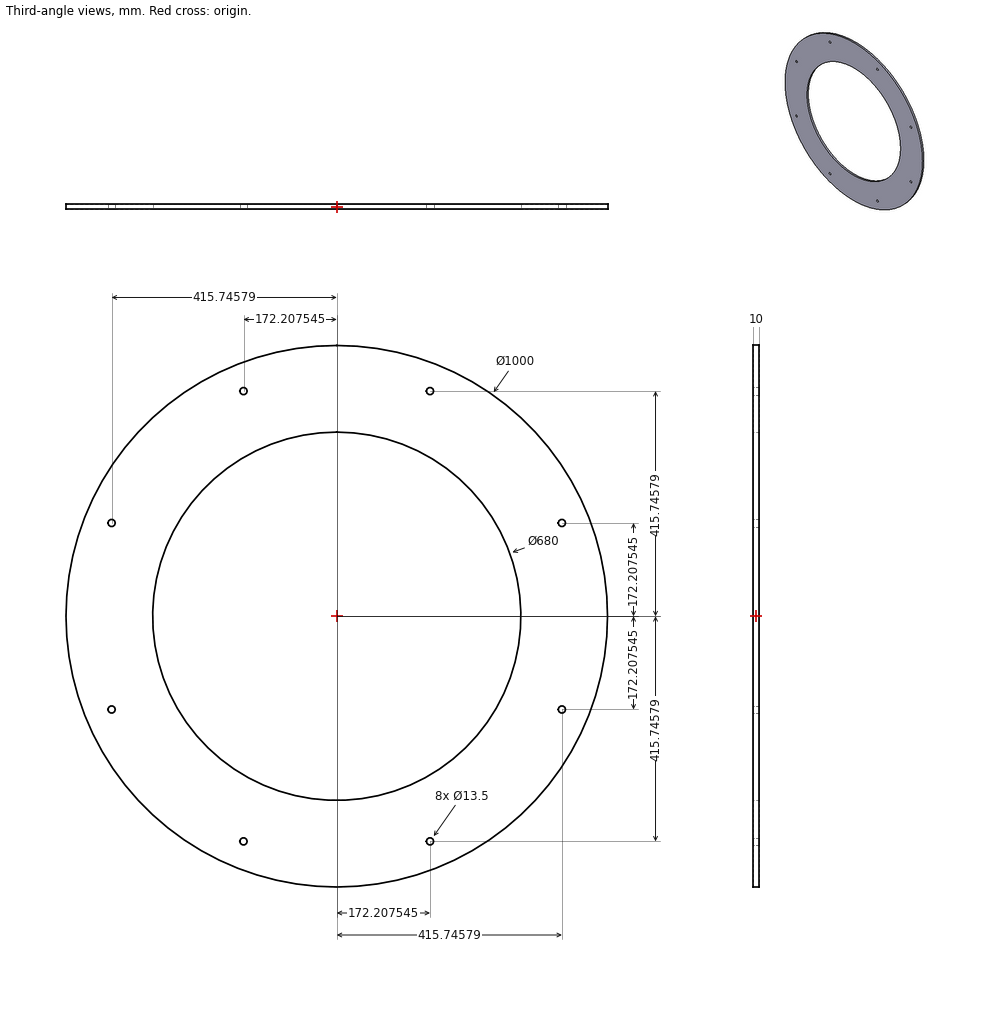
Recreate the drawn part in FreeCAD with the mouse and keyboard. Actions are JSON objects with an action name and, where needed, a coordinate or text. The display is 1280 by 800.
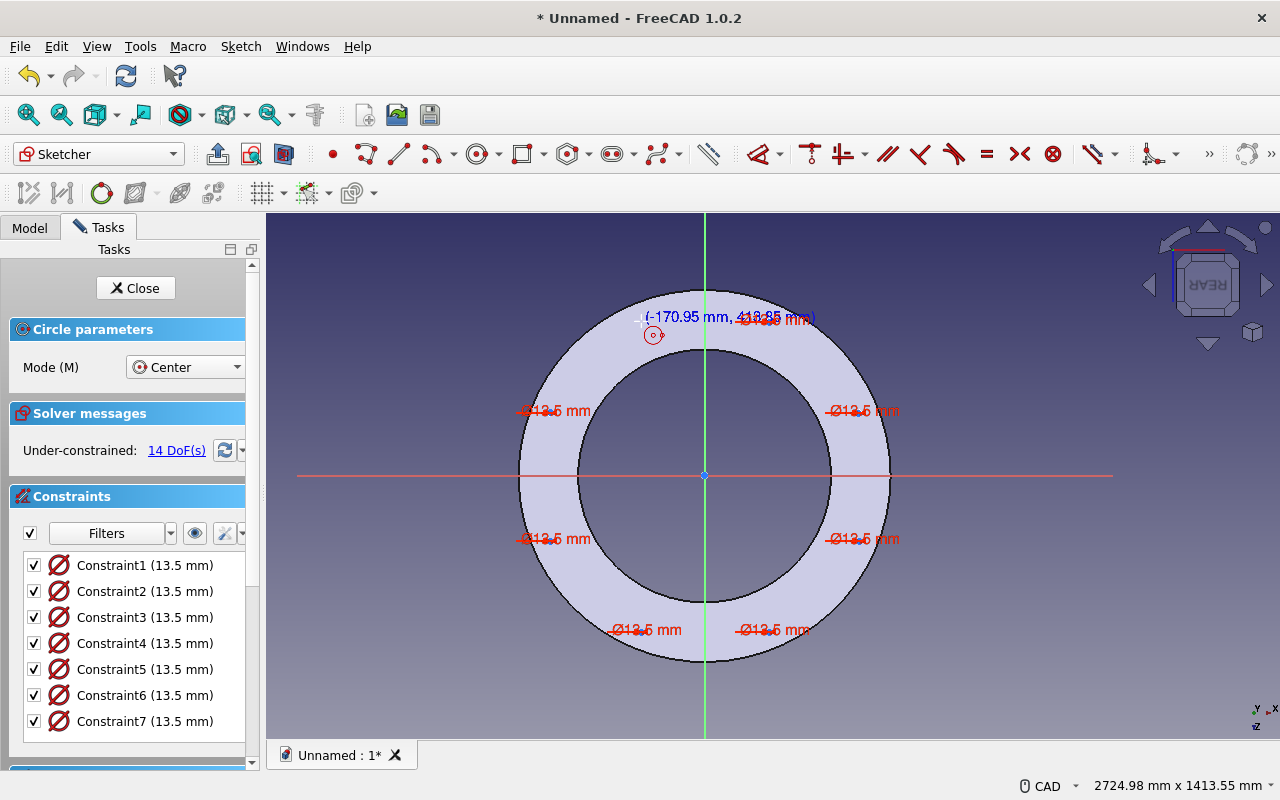
{"action": "left_click", "coordinate": [641, 321]}
{"action": "mouse_move", "coordinate": [642, 320]}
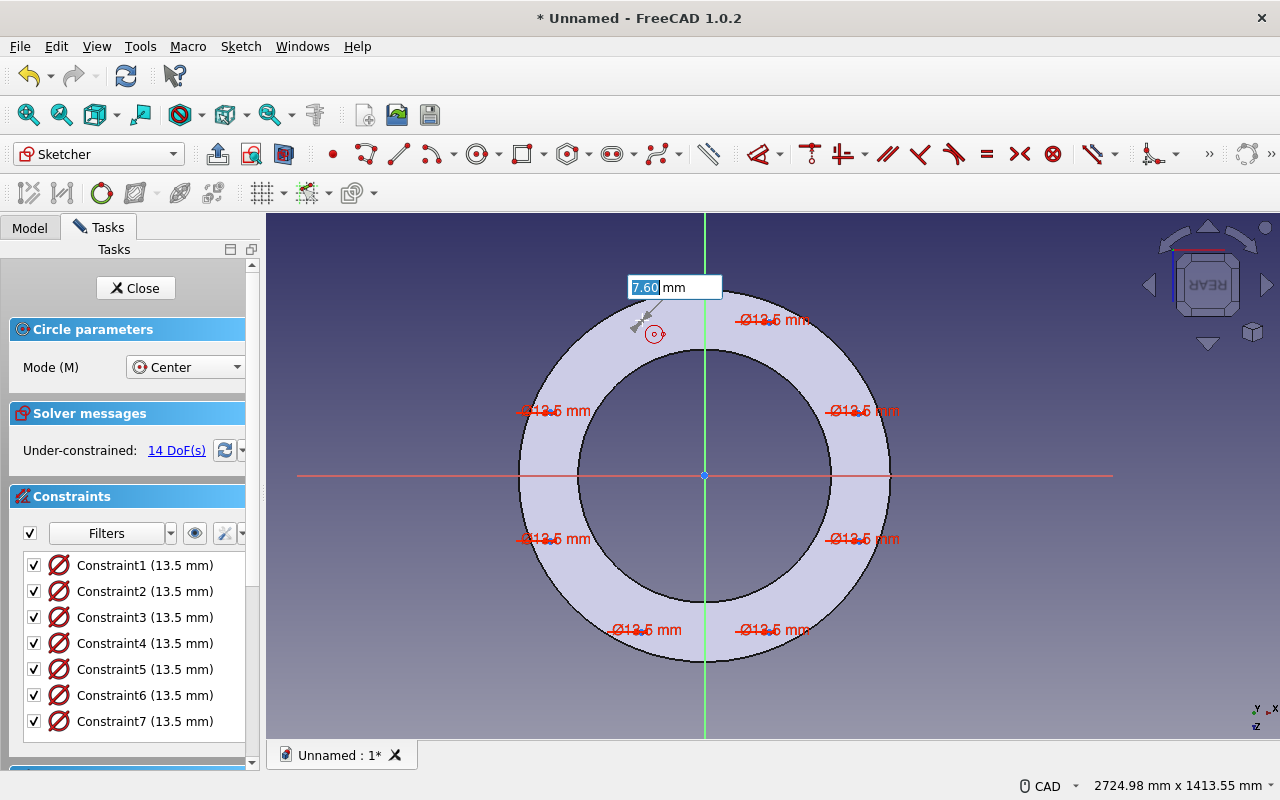
{"action": "type", "text": "13.5"}
{"action": "key", "text": "Return"}
{"action": "key", "text": "Escape"}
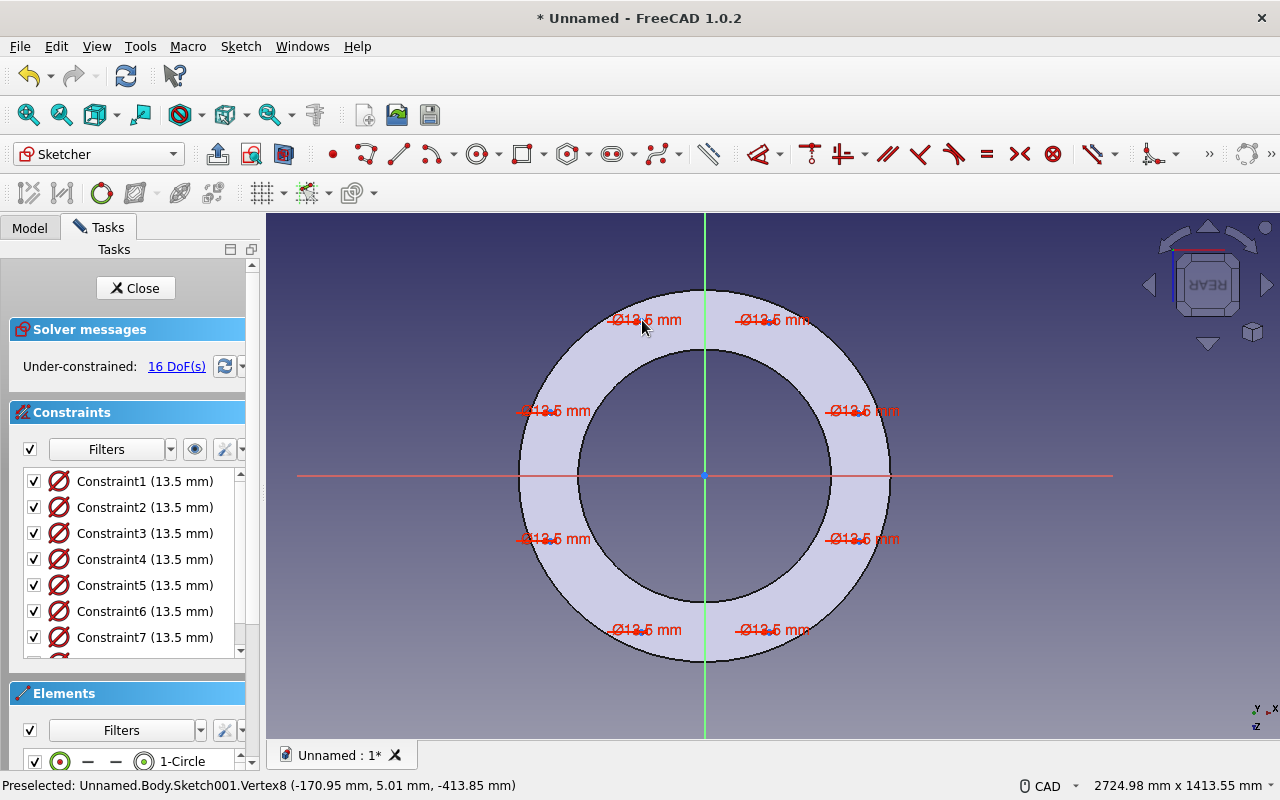
{"action": "left_click", "coordinate": [859, 413]}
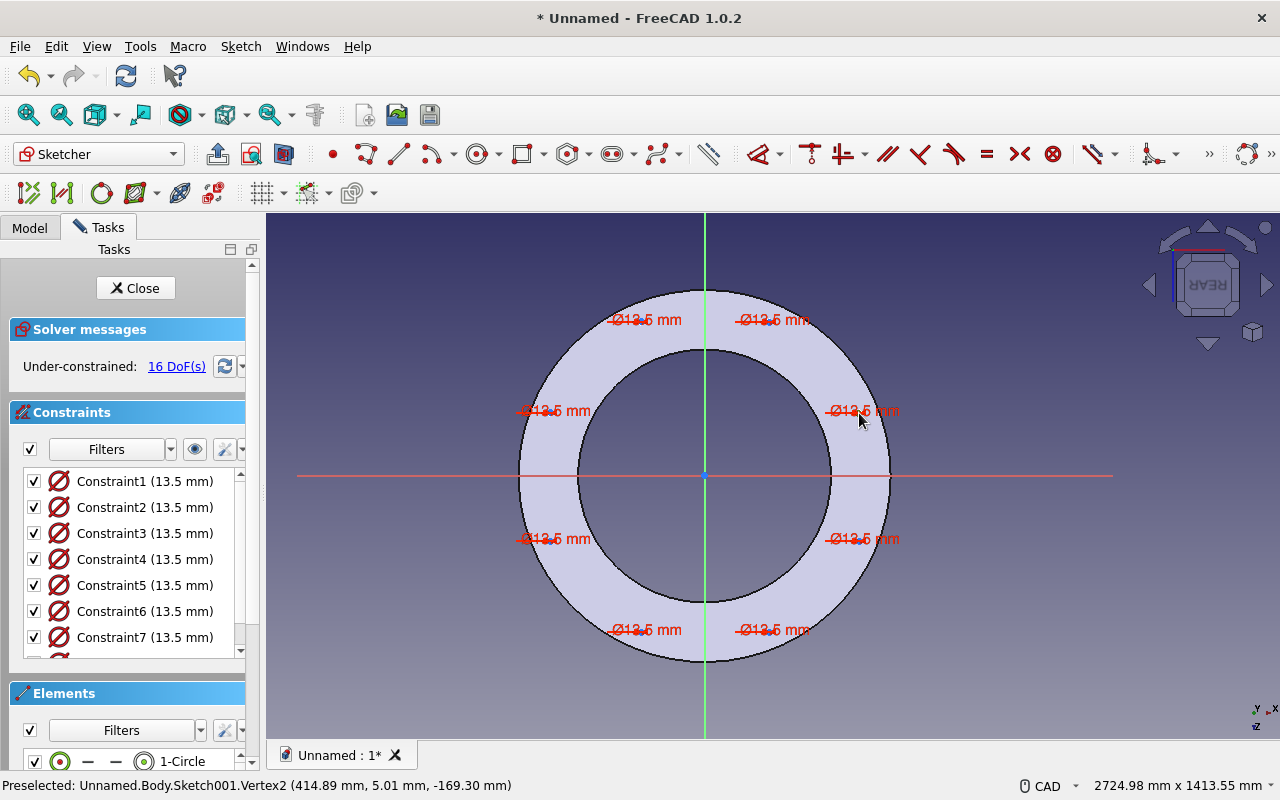
{"action": "left_click", "coordinate": [859, 541]}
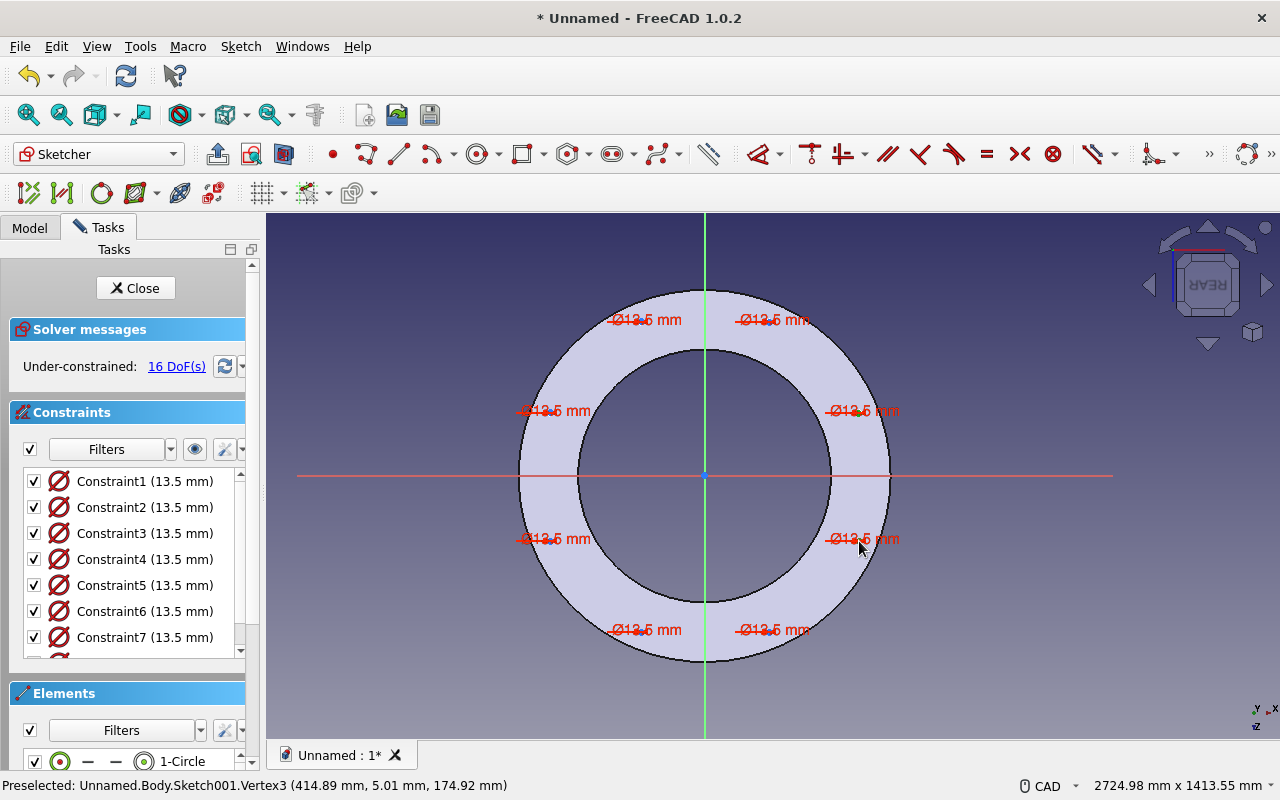
{"action": "key", "text": "v"}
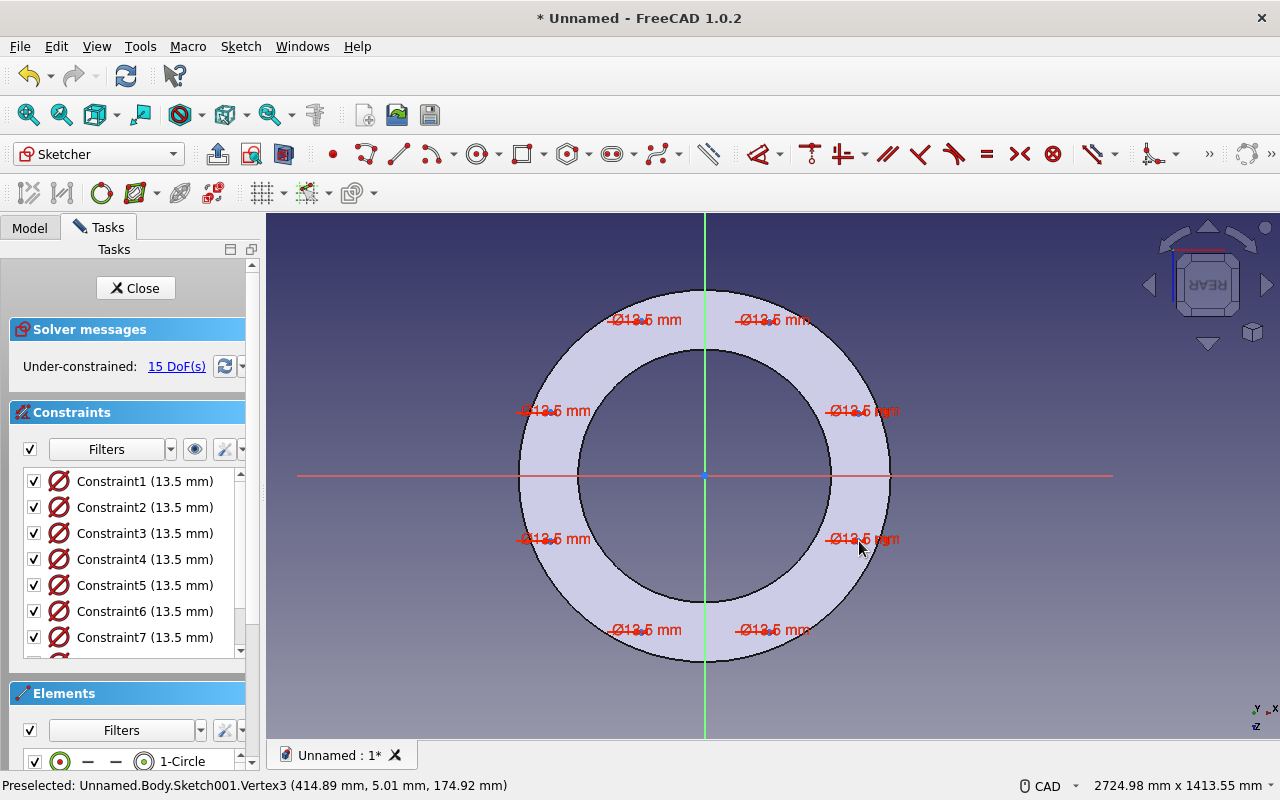
{"action": "left_click", "coordinate": [769, 322]}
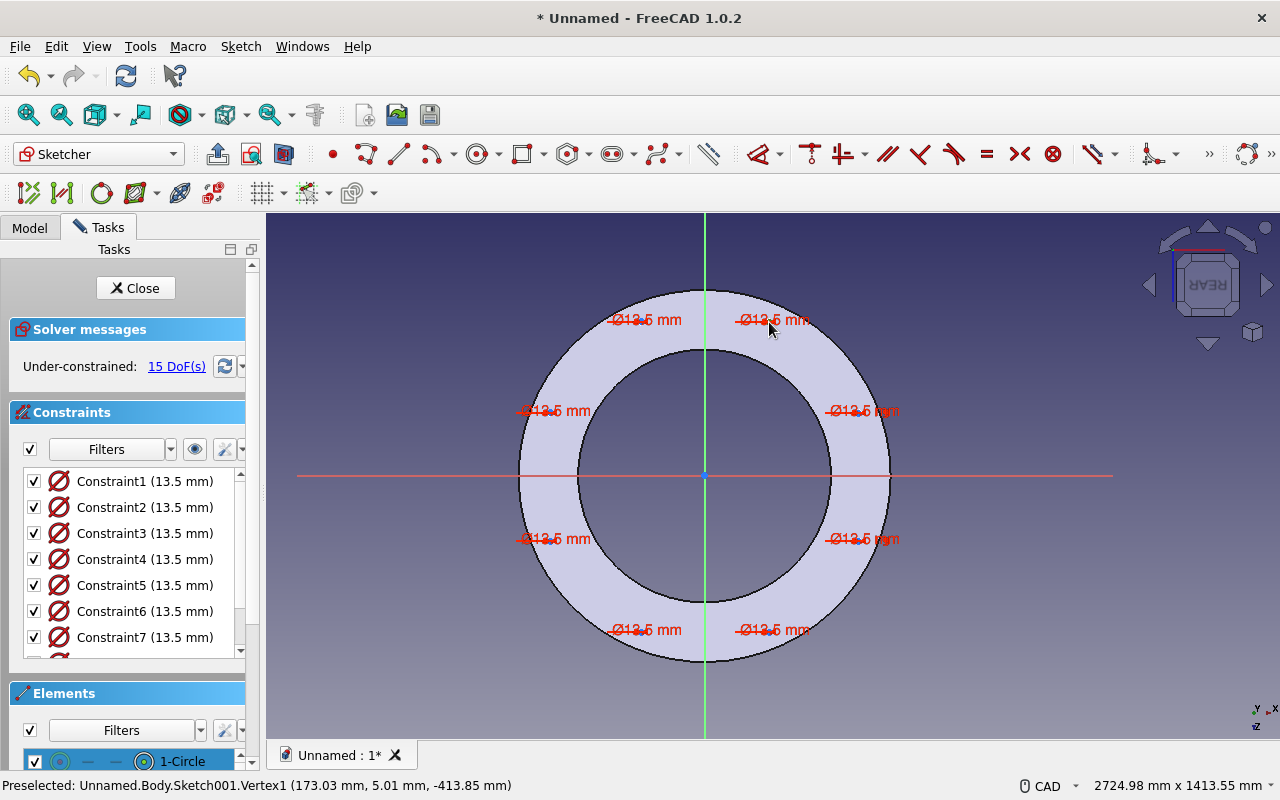
{"action": "left_click", "coordinate": [769, 632]}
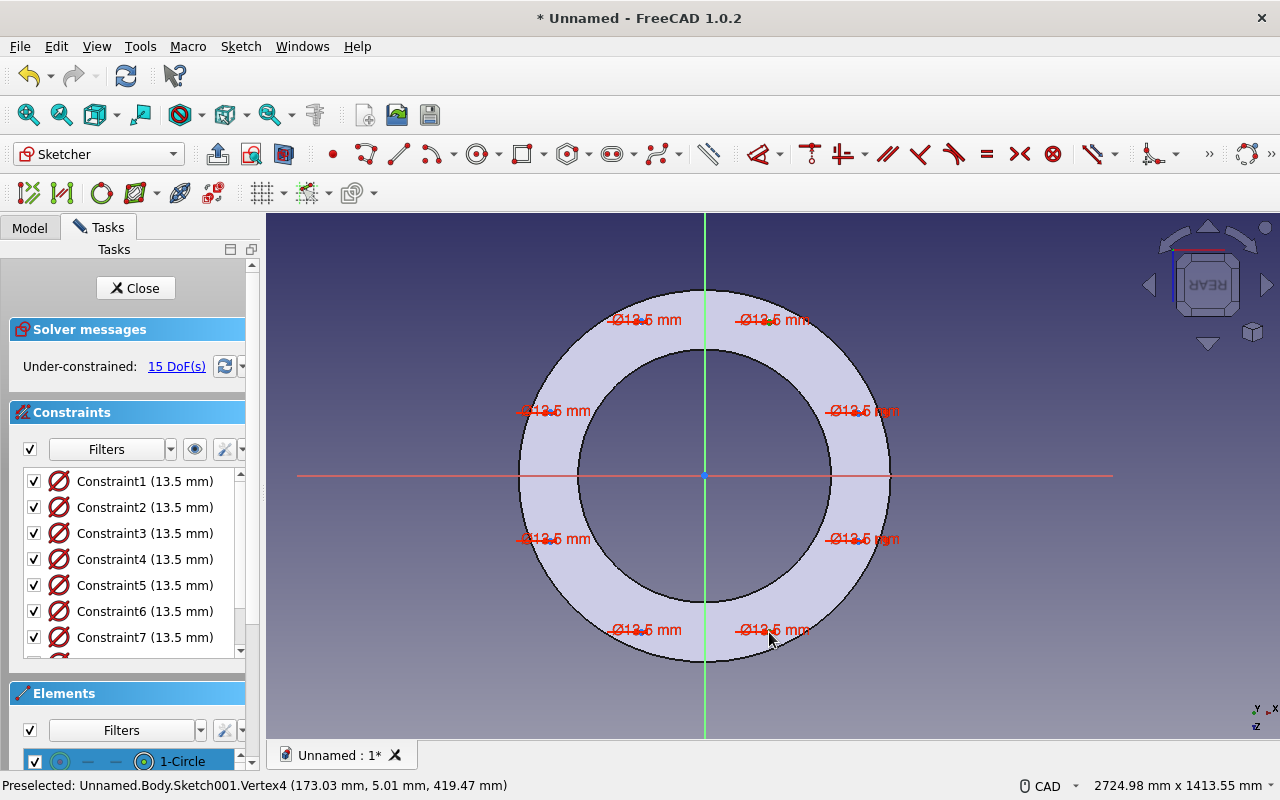
{"action": "key", "text": "v"}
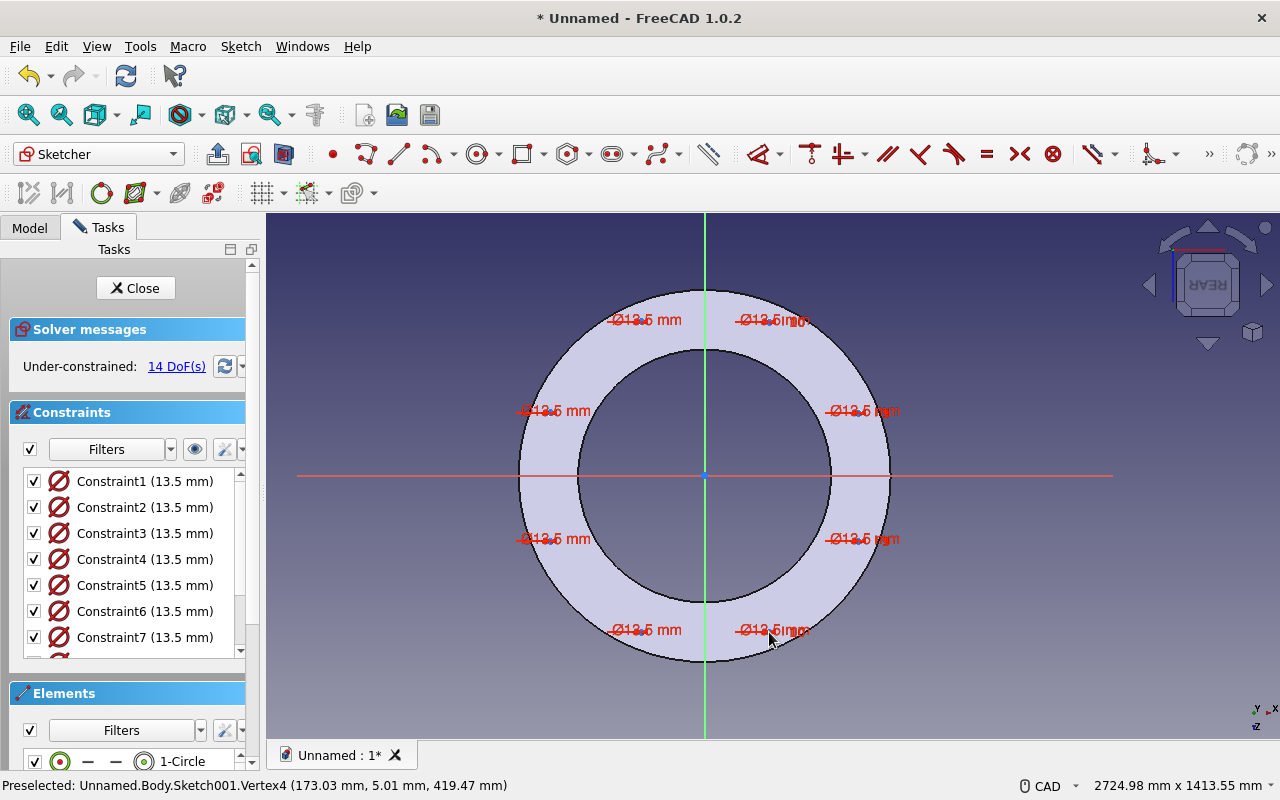
{"action": "left_click", "coordinate": [769, 632]}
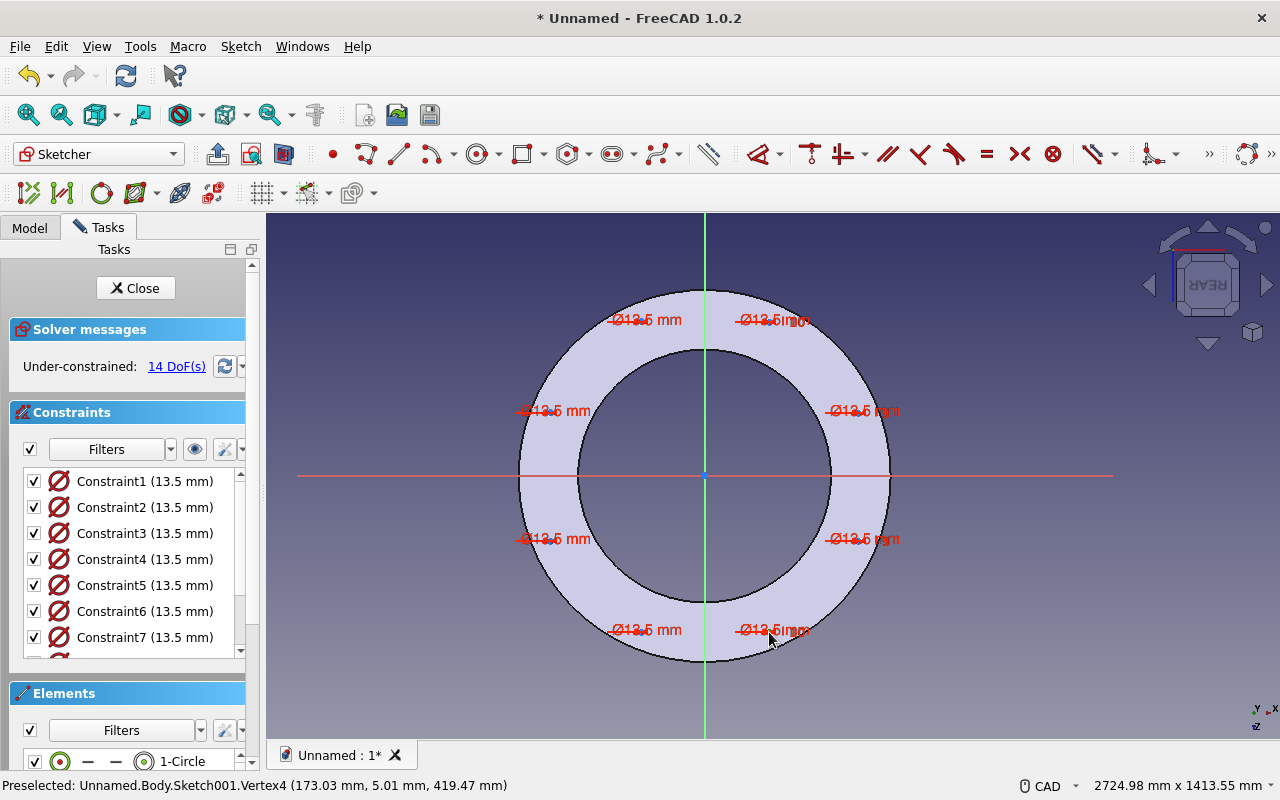
{"action": "left_click", "coordinate": [641, 632]}